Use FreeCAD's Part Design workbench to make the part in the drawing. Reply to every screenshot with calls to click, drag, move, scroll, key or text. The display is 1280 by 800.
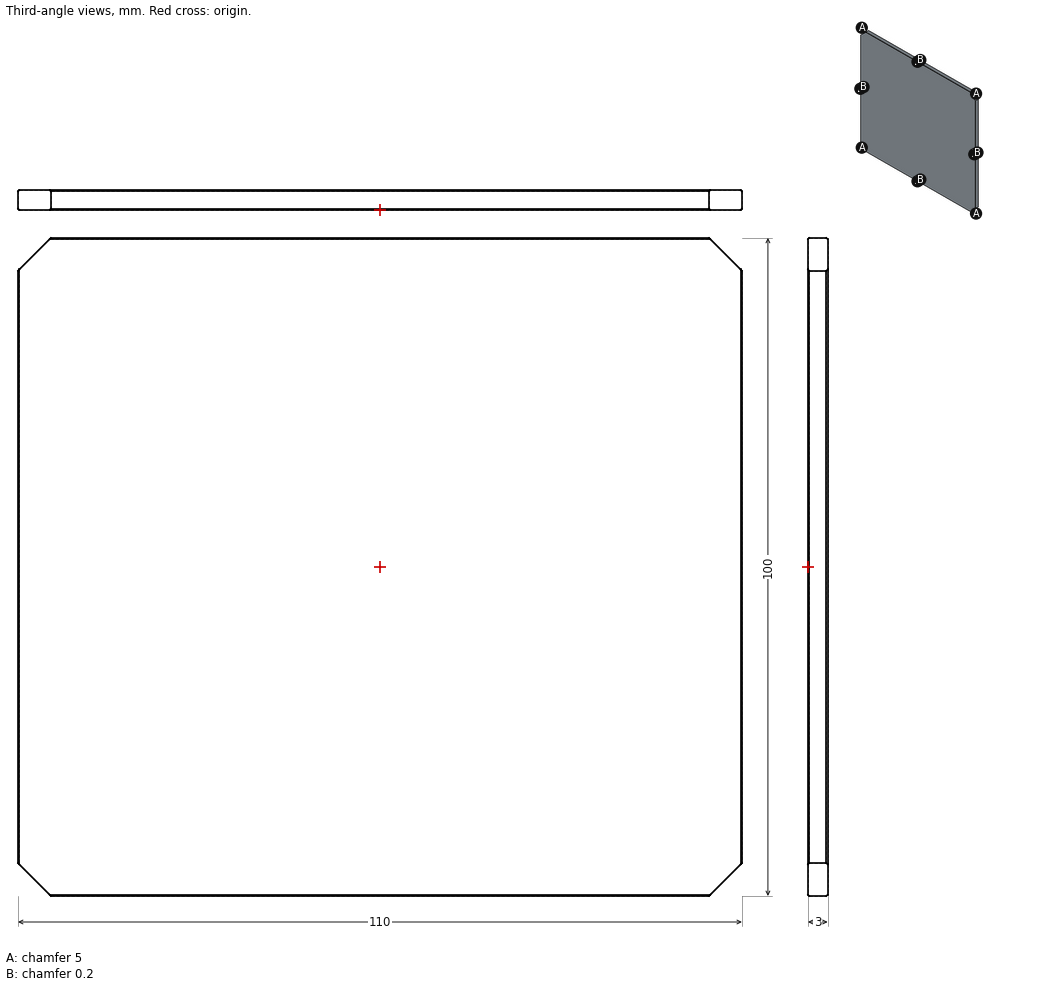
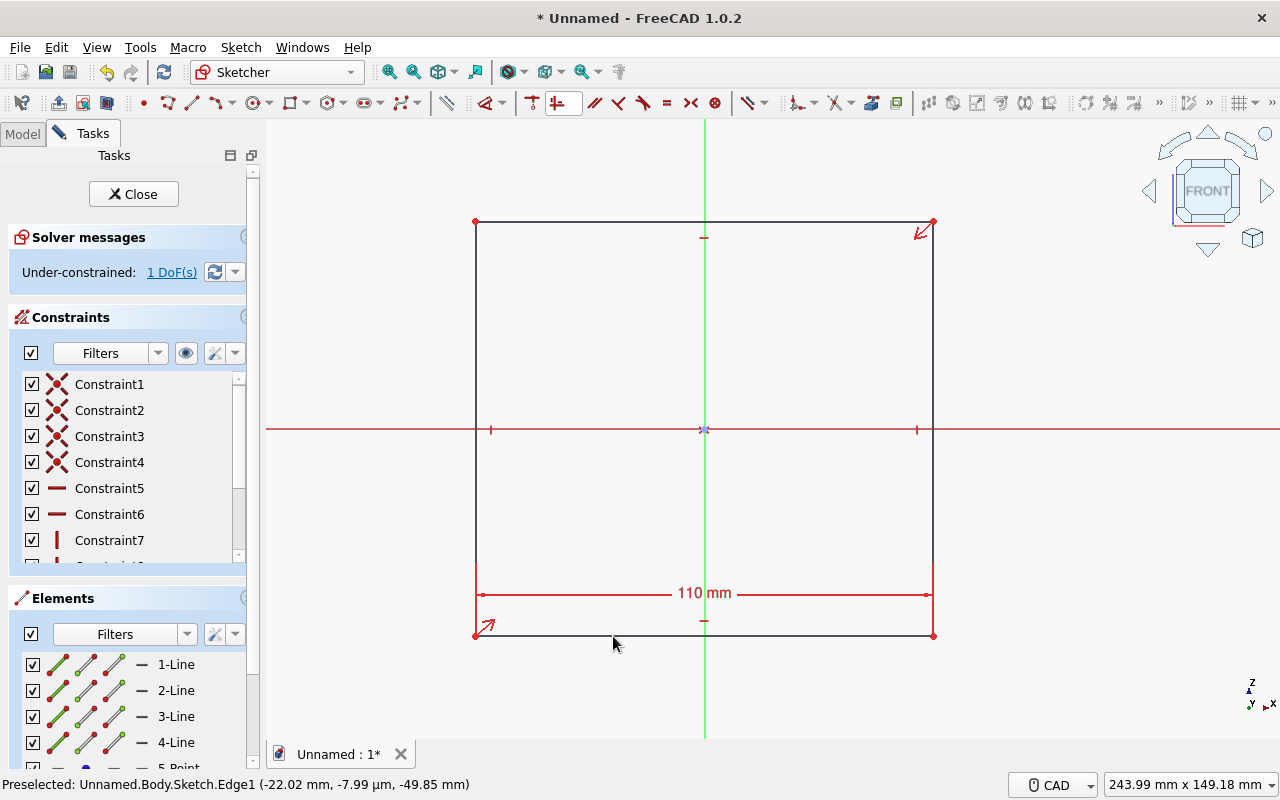
click(933, 512)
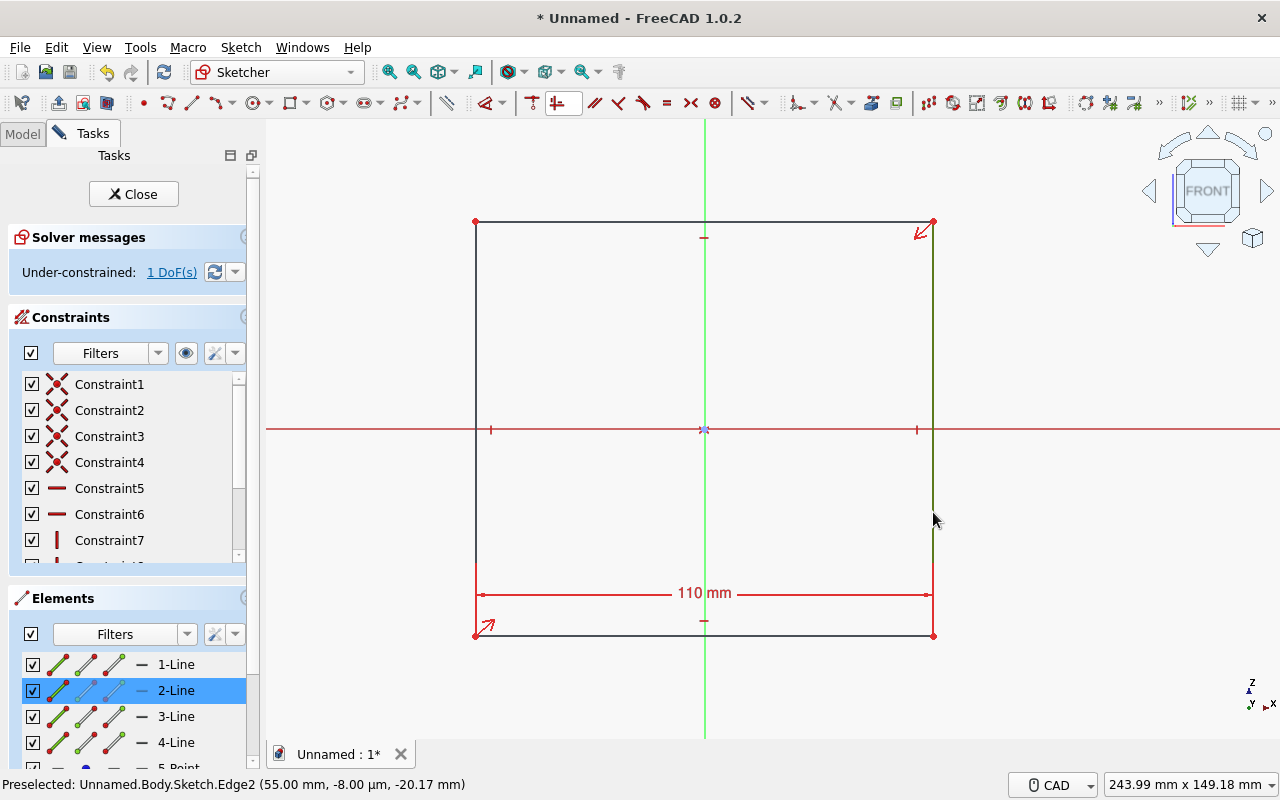
key(i)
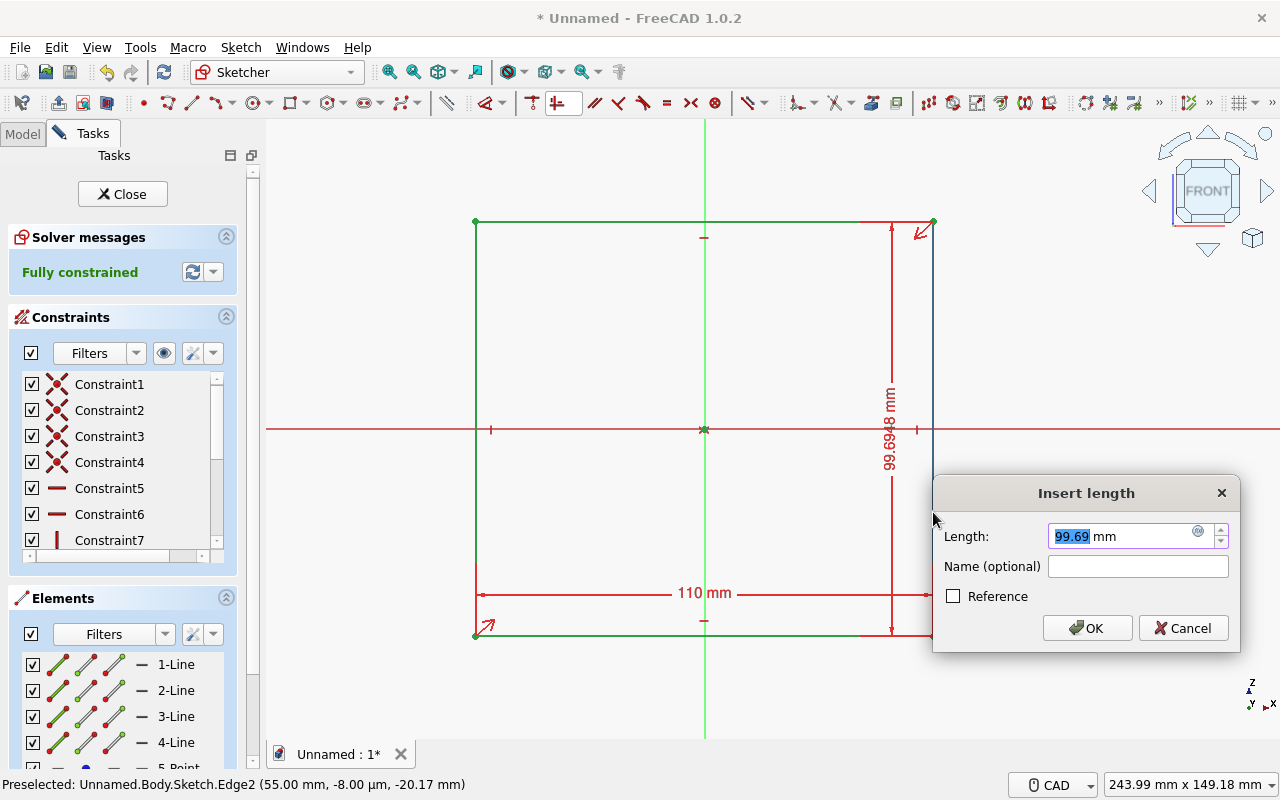
text(100)
key(Return)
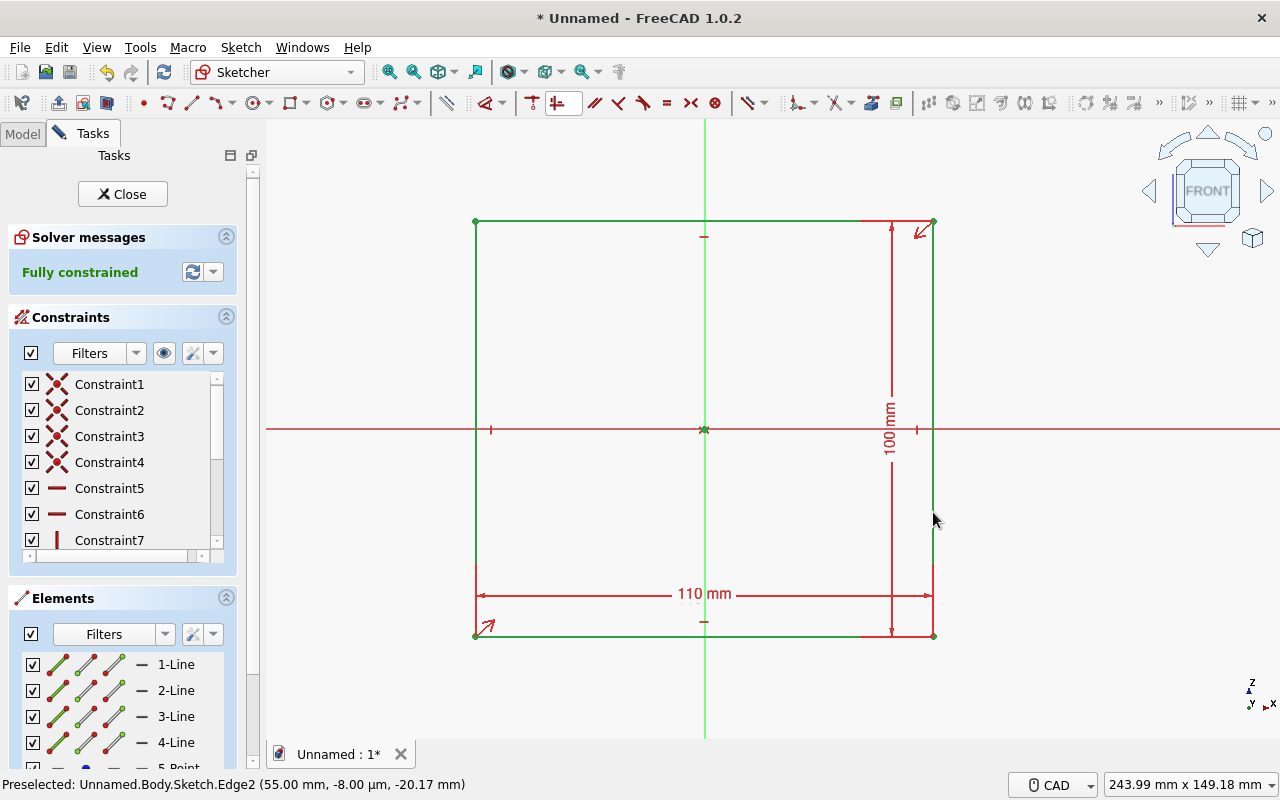
click(123, 194)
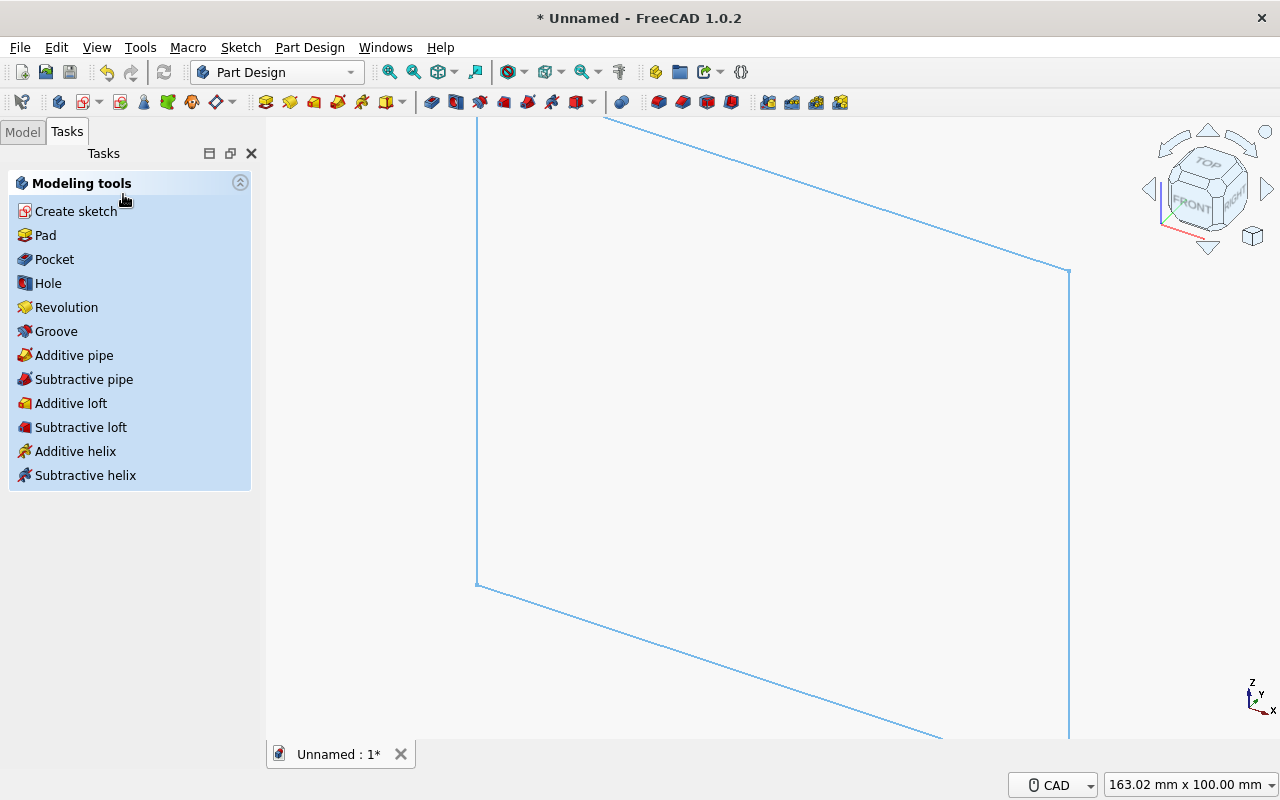
click(266, 102)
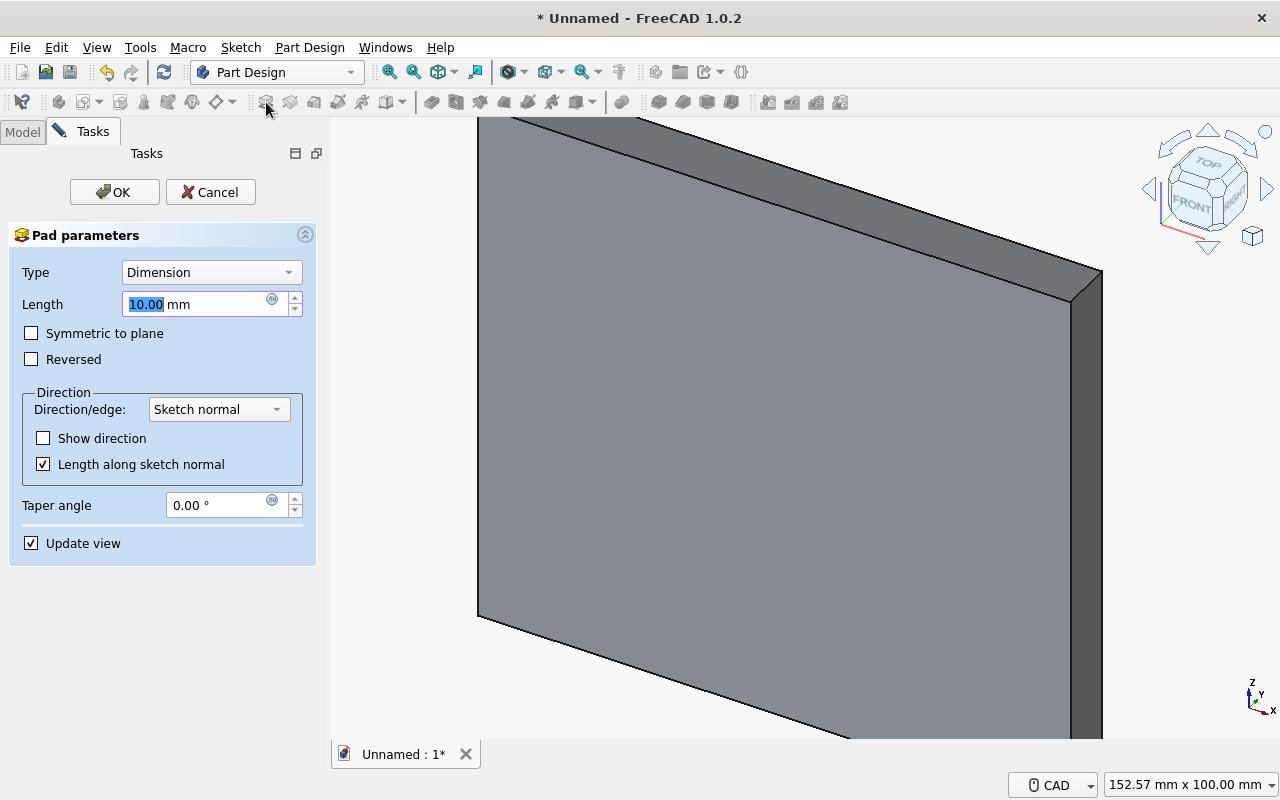
text(3)
key(Tab)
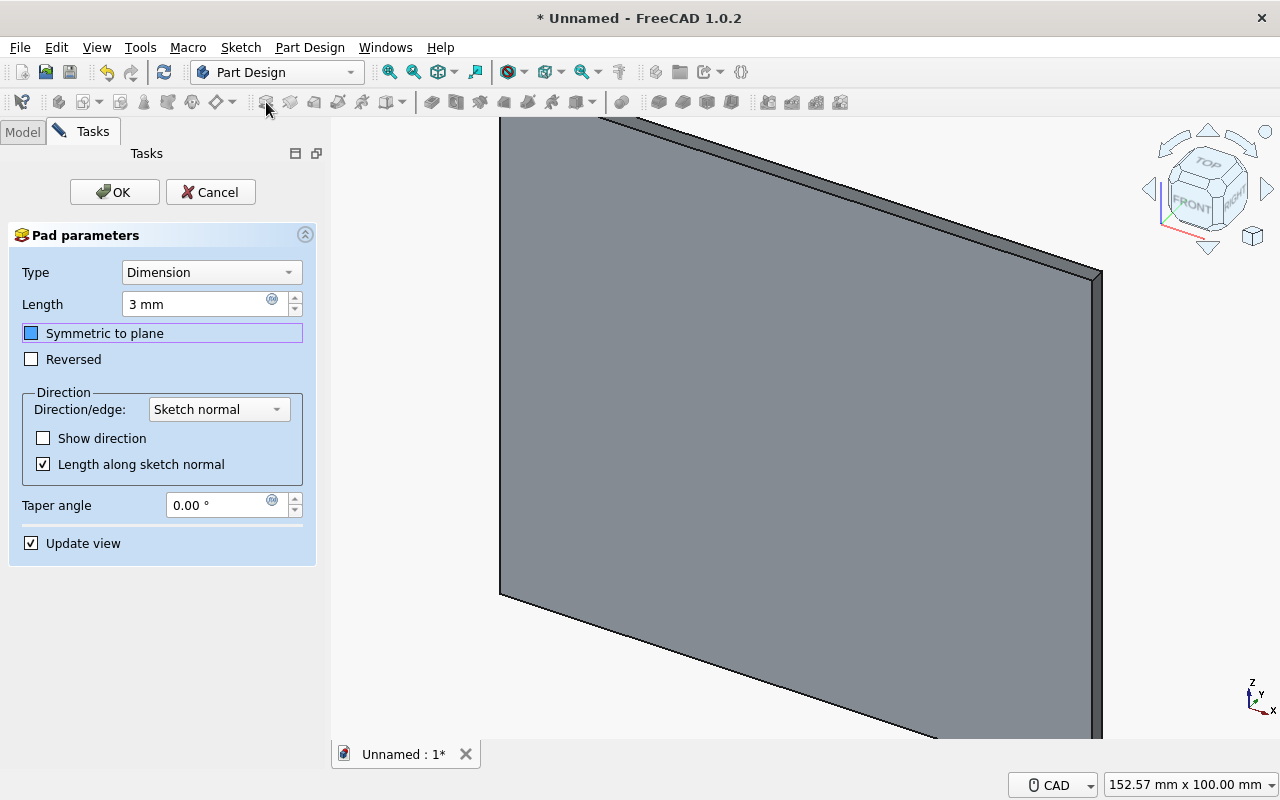
click(30, 359)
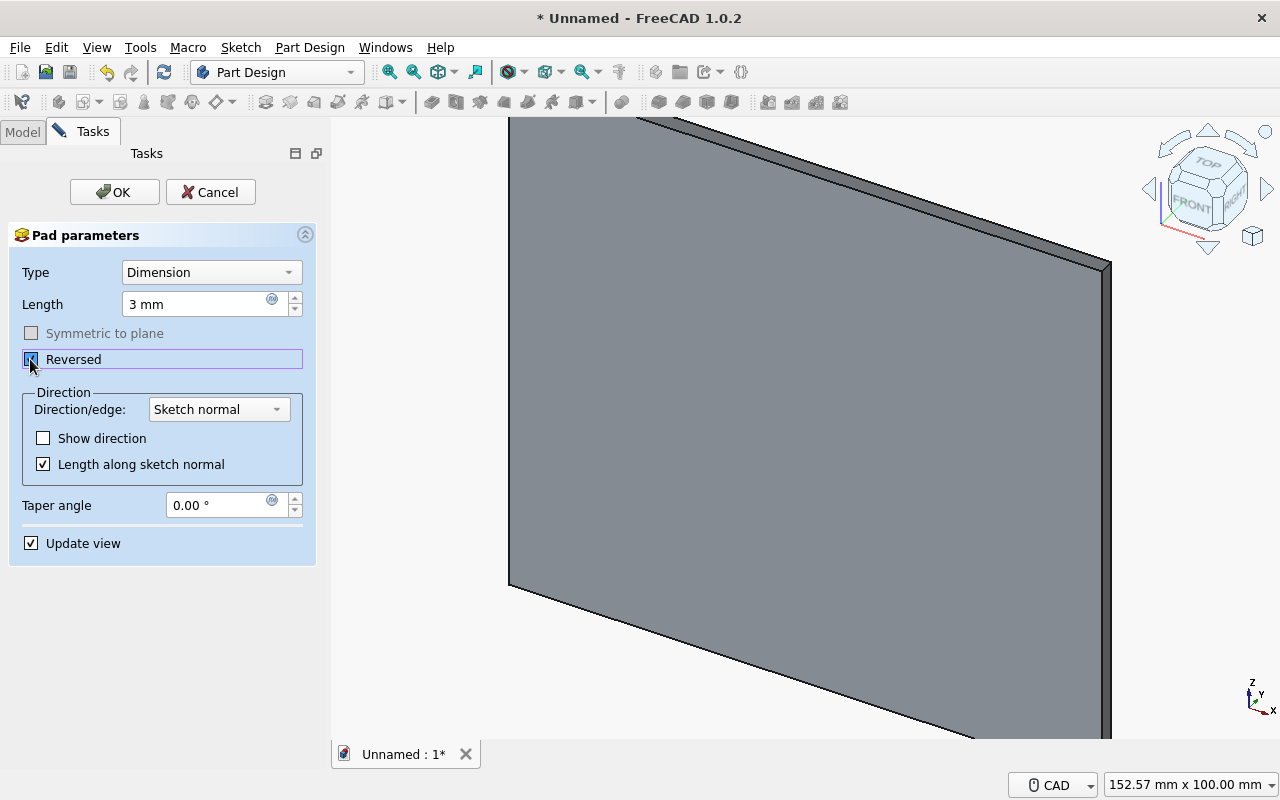
click(115, 192)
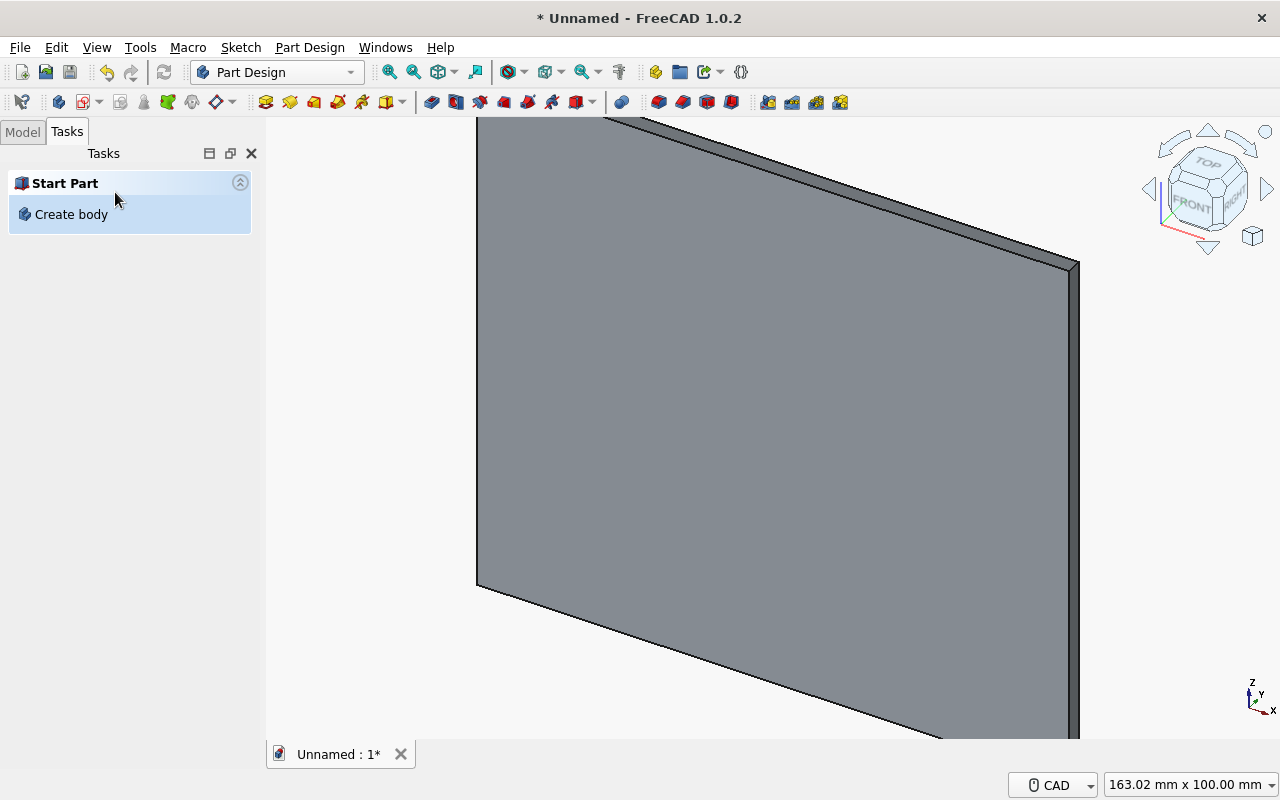
click(390, 72)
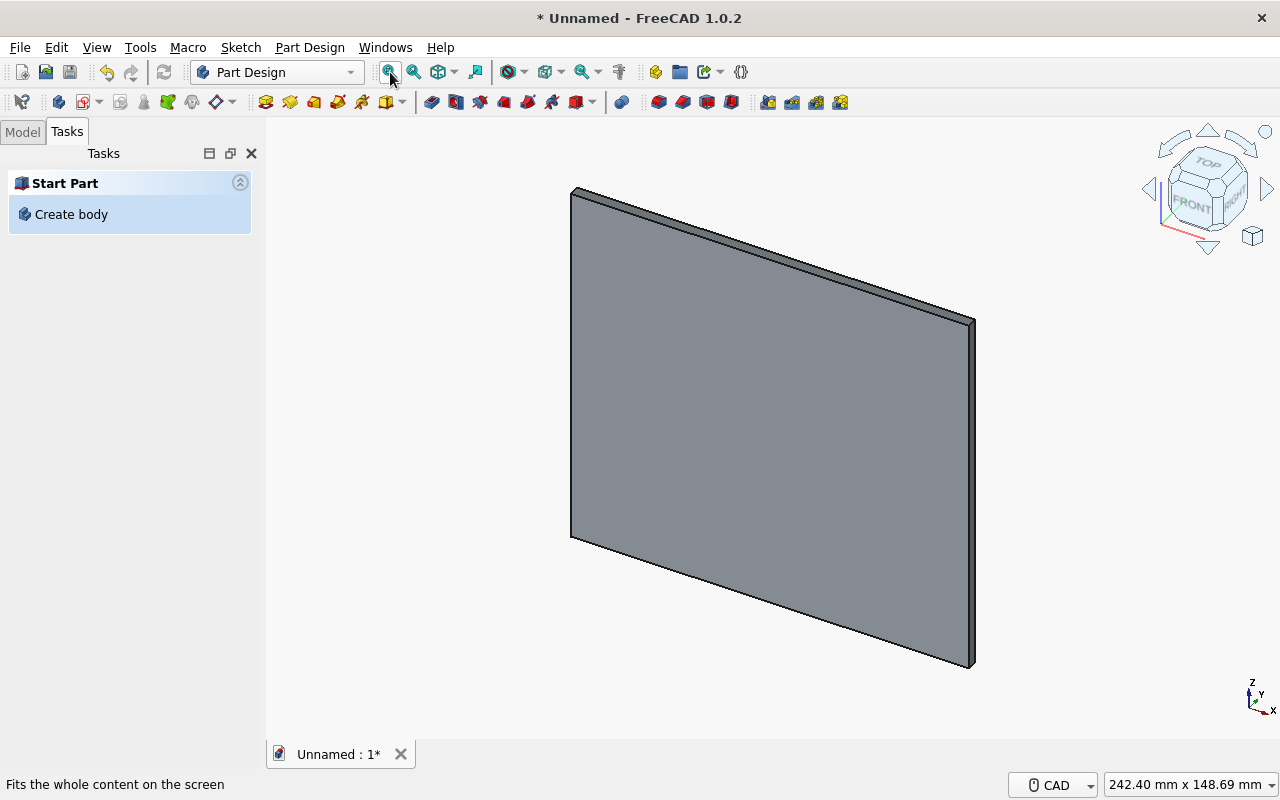
click(974, 320)